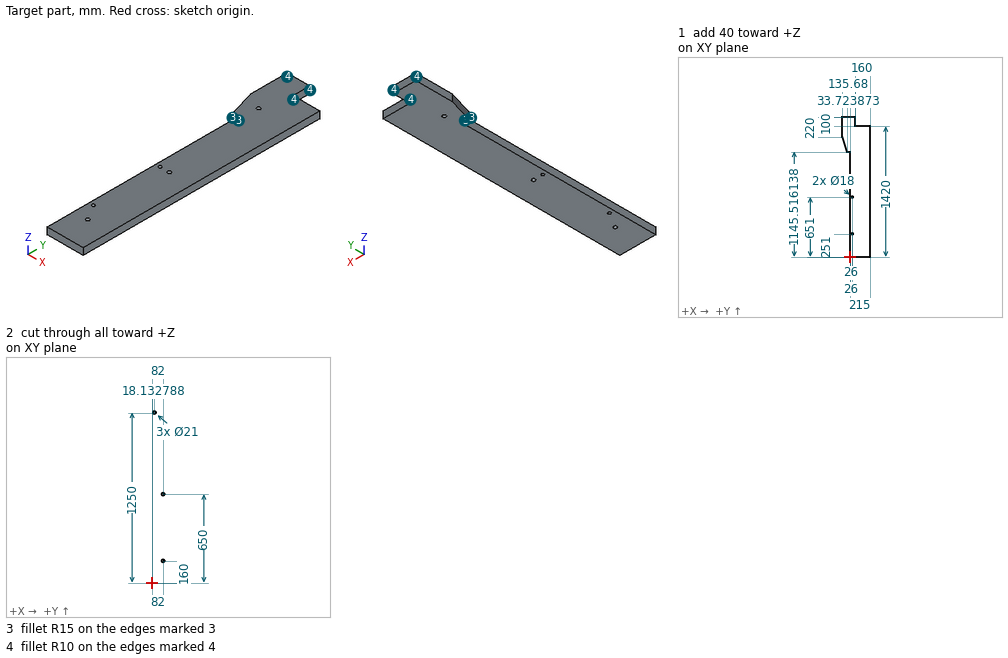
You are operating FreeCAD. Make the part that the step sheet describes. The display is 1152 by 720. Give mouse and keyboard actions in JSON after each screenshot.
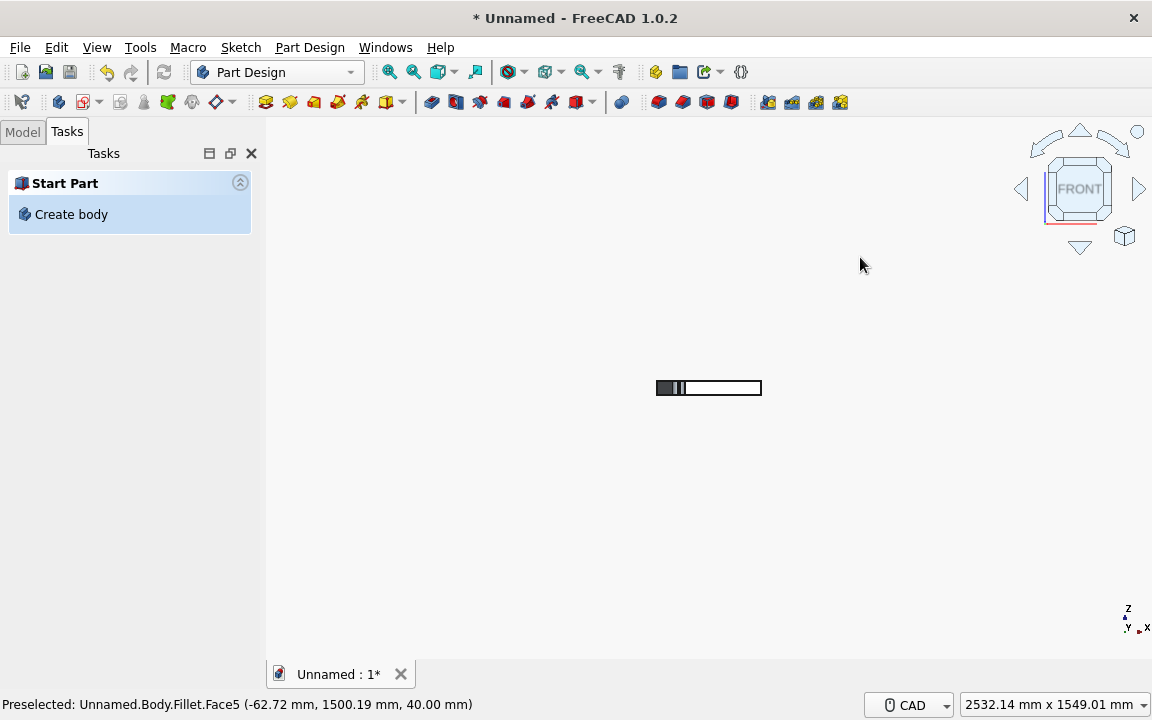
{"action": "key", "text": "v f"}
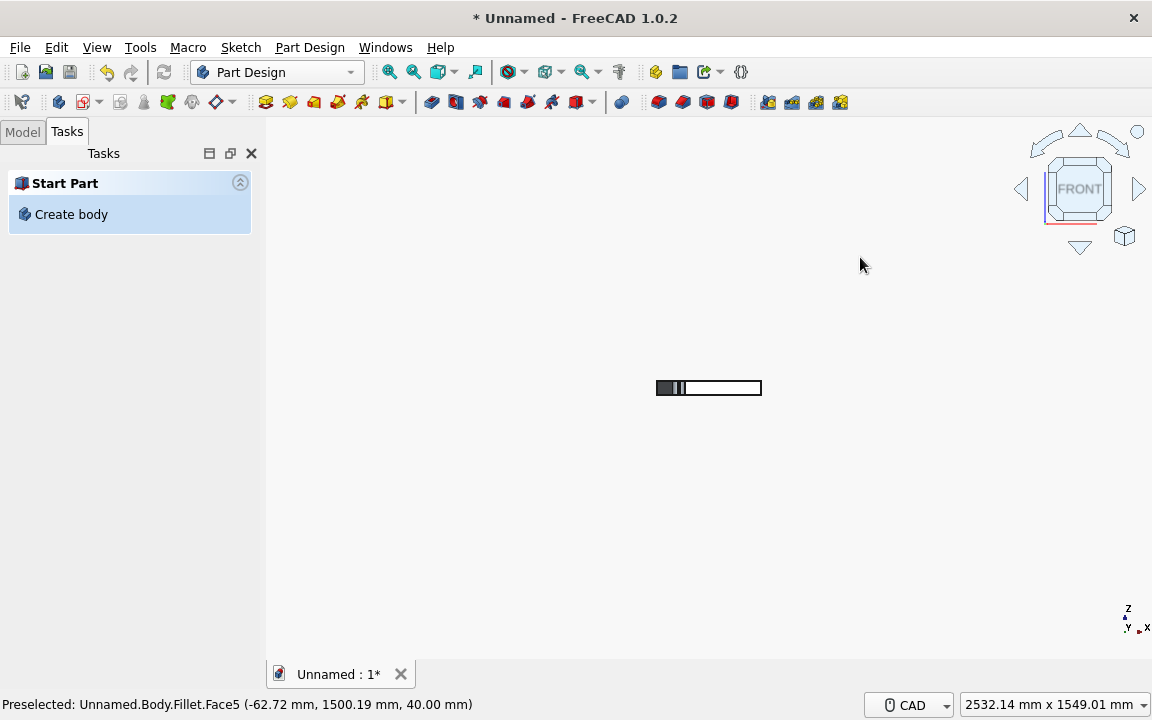
{"action": "scroll", "coordinate": [657, 387], "scroll_direction": "up", "scroll_amount": 6}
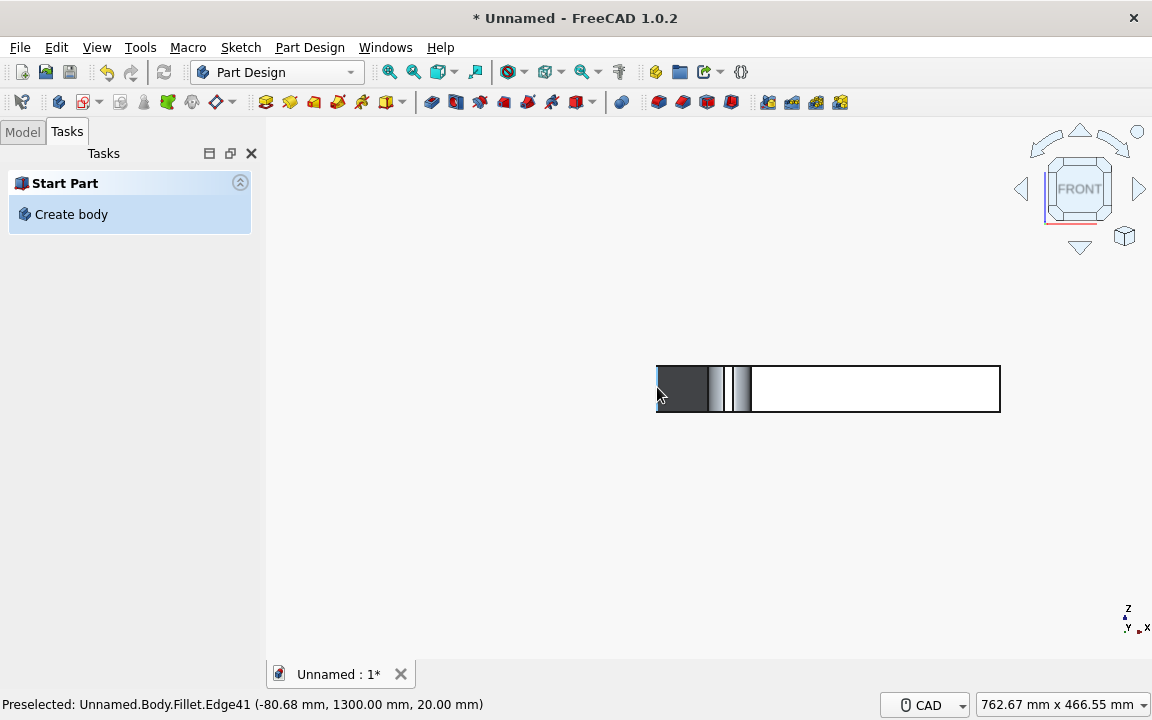
{"action": "key", "text": "v f"}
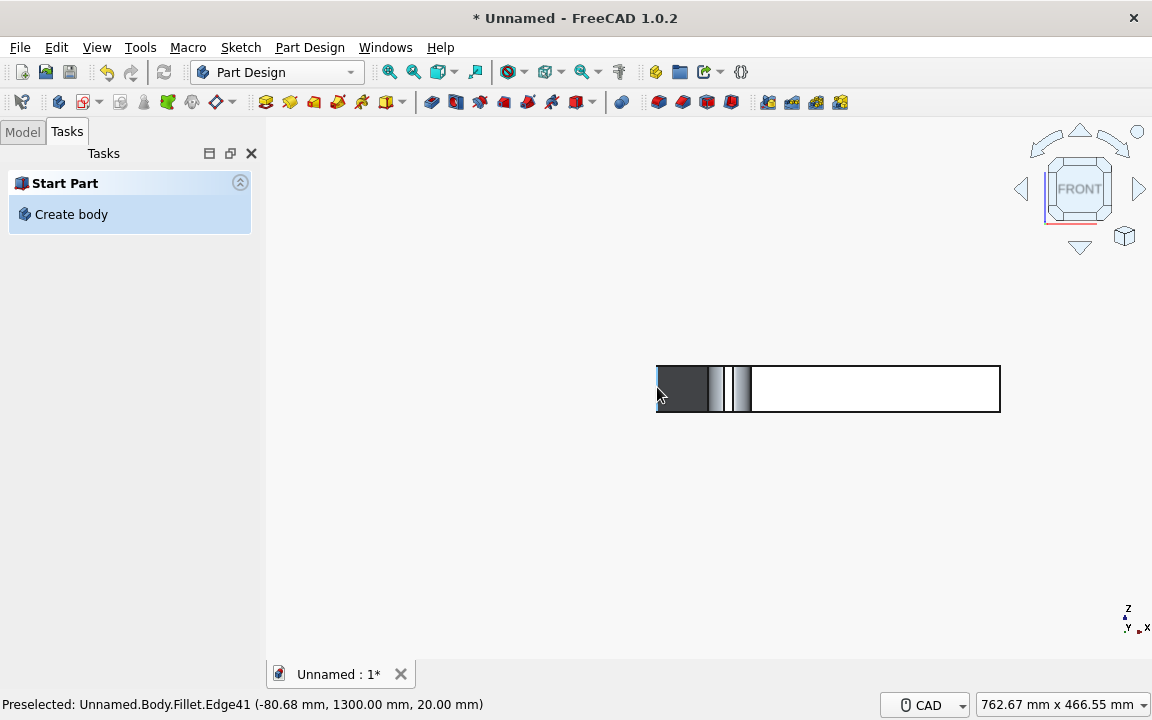
{"action": "key", "text": "3"}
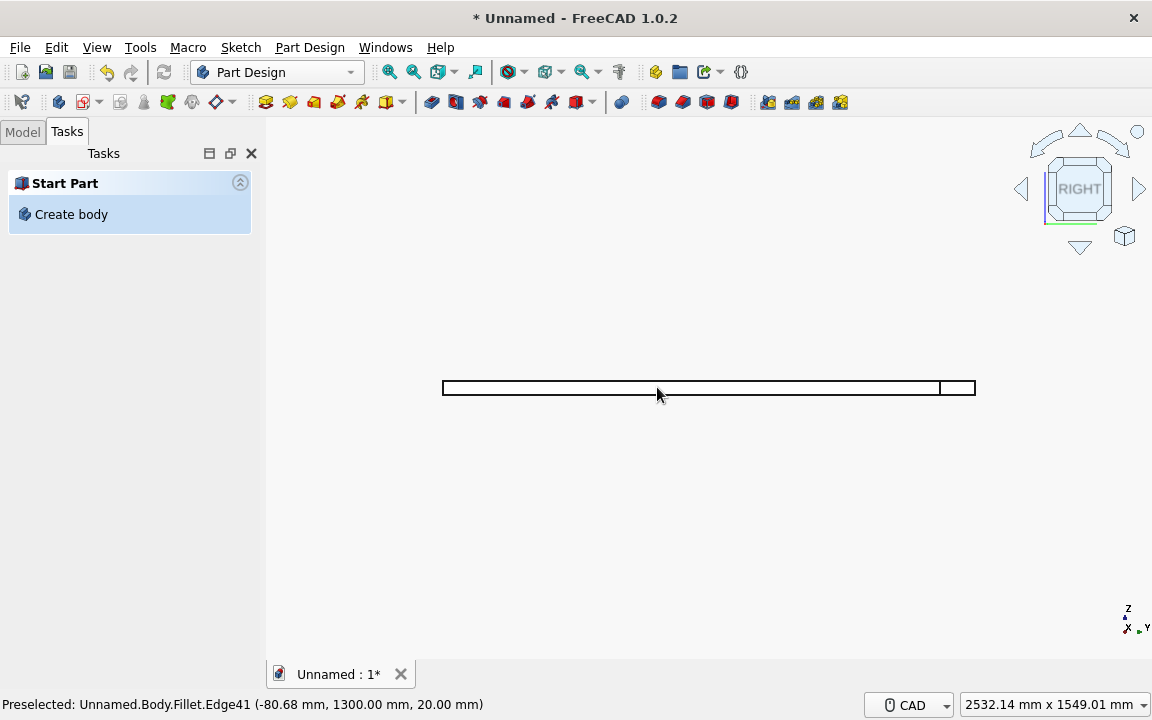
{"action": "left_click", "coordinate": [975, 387]}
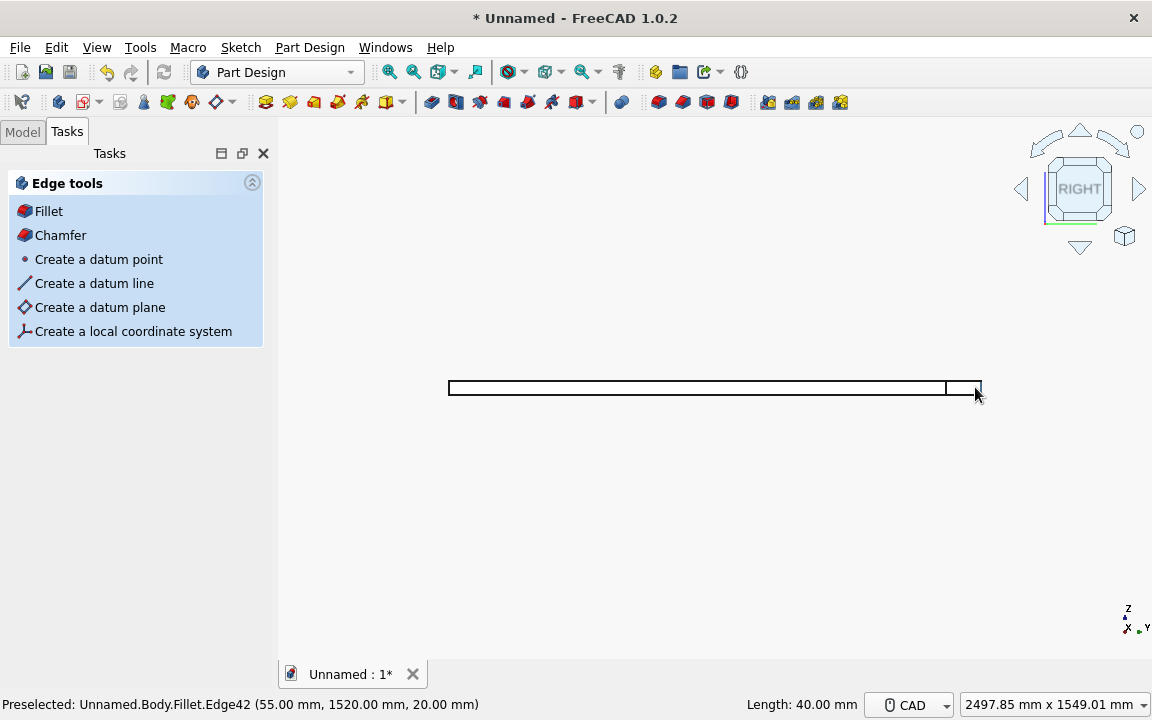
{"action": "scroll", "coordinate": [981, 387], "scroll_direction": "up", "scroll_amount": 6}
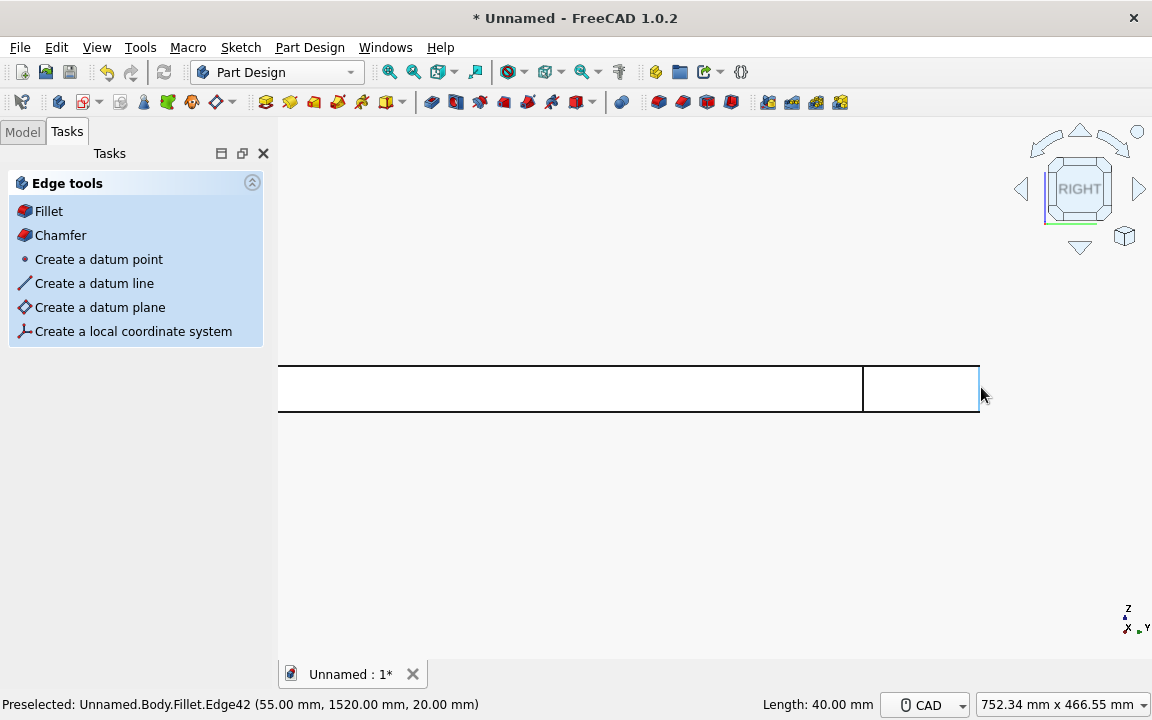
{"action": "key", "text": "v f"}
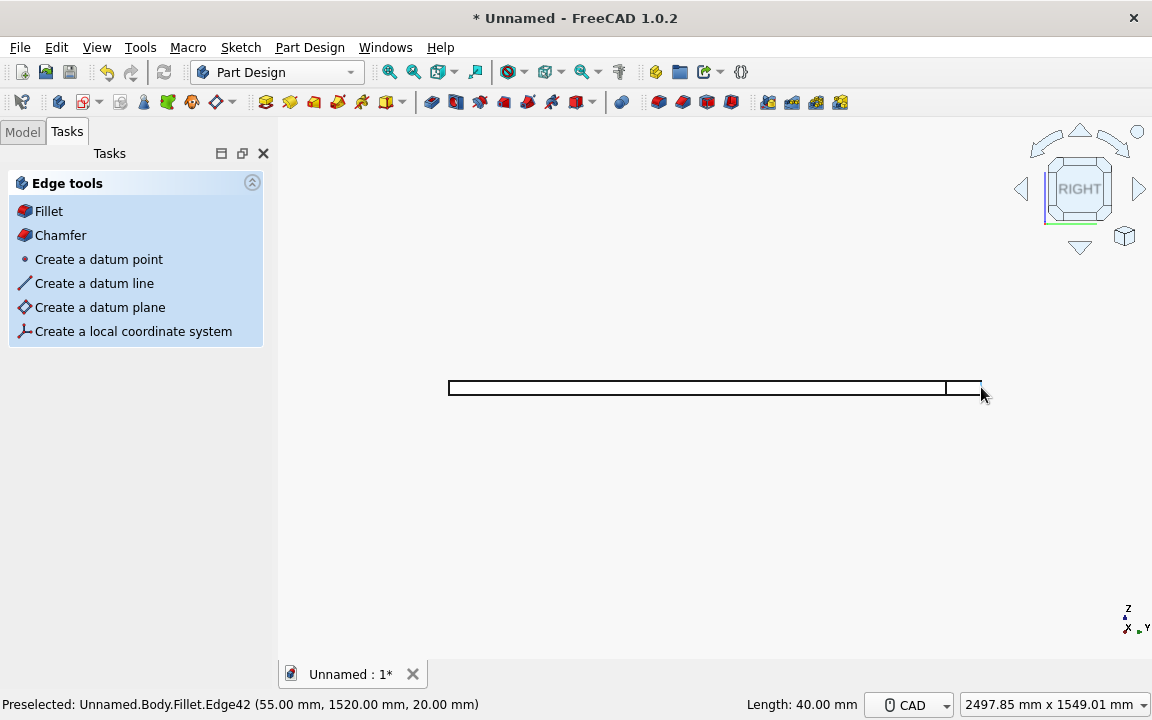
{"action": "key", "text": "5"}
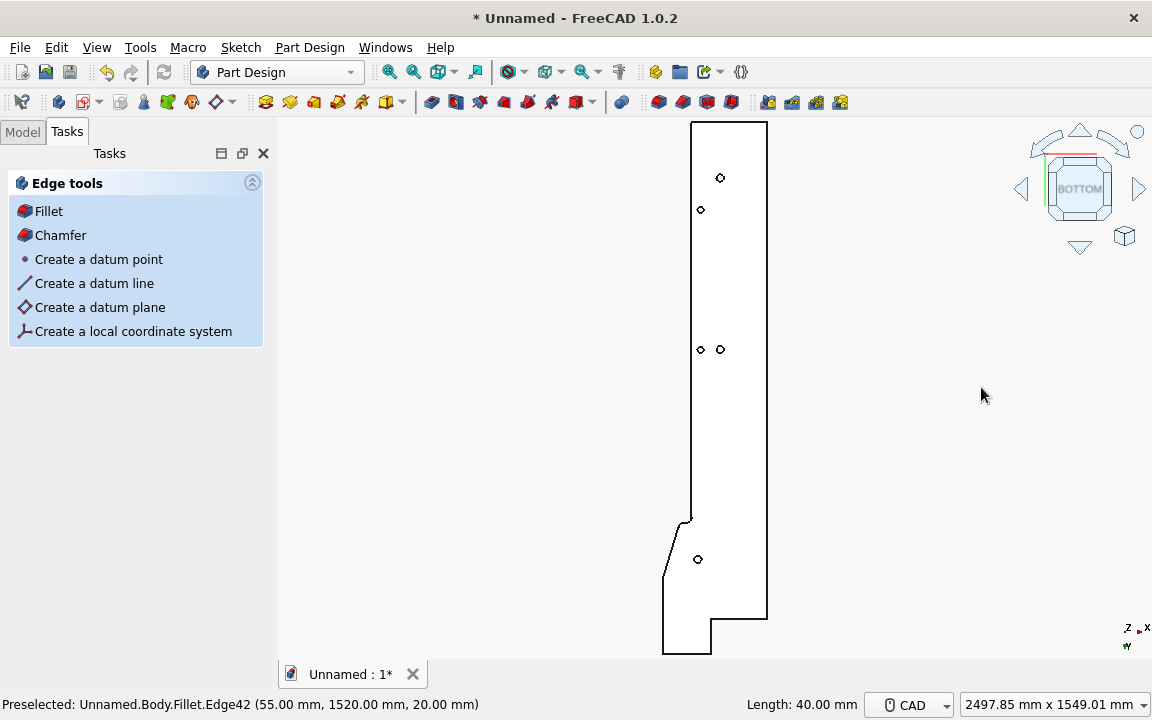
{"action": "key", "text": "4"}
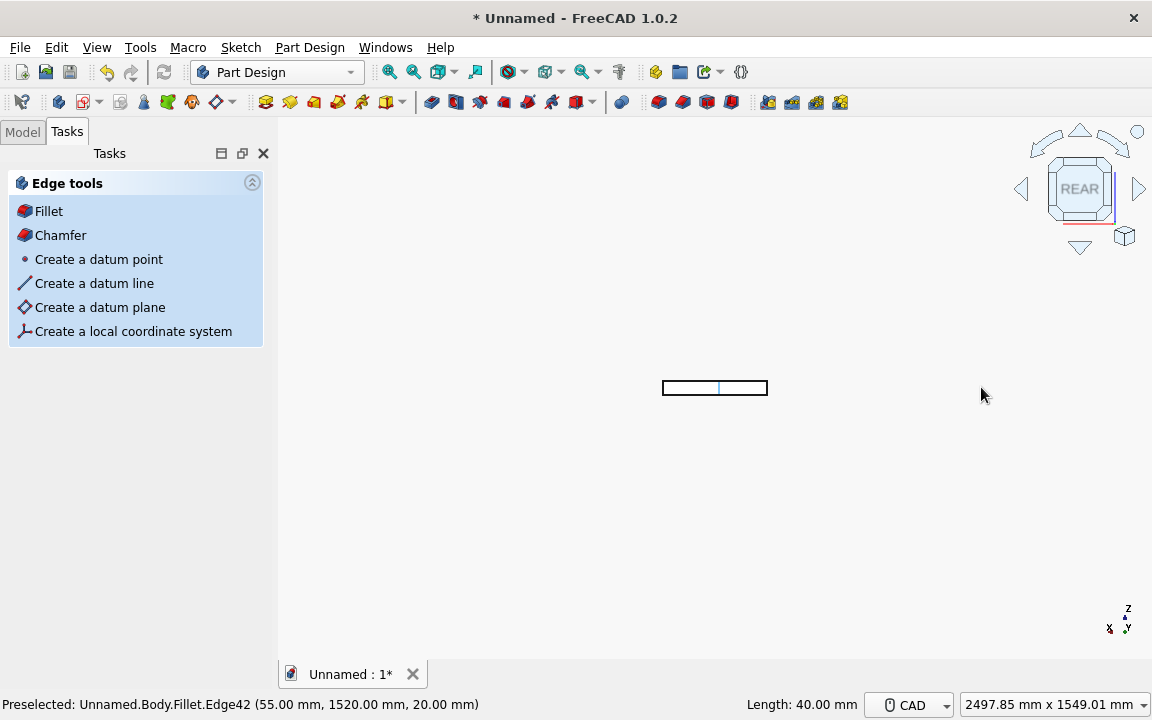
{"action": "key", "text": "v f"}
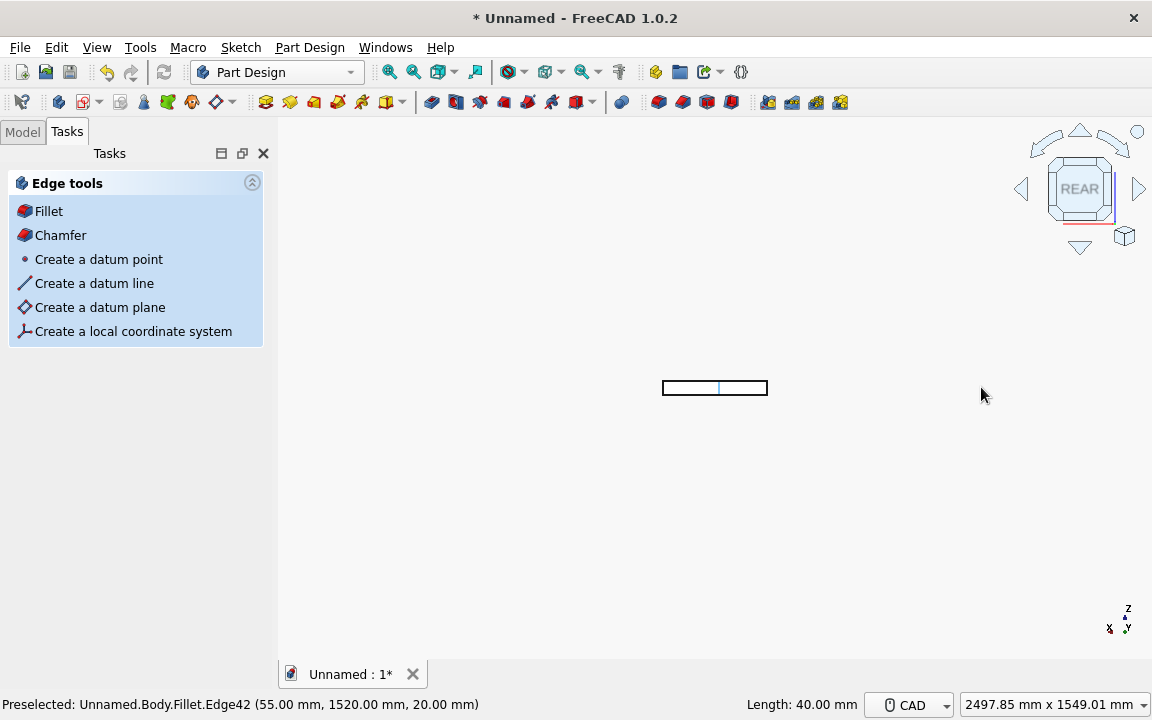
{"action": "left_click", "coordinate": [767, 387], "text": "ctrl"}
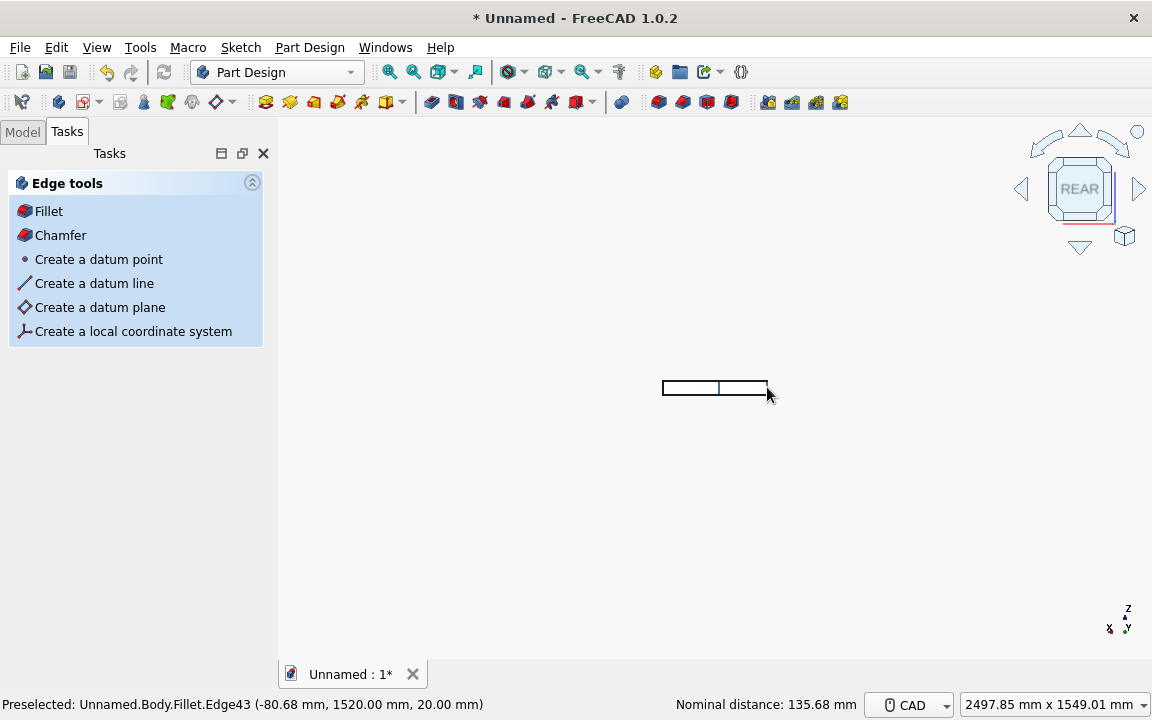
{"action": "scroll", "coordinate": [719, 387], "scroll_direction": "up", "scroll_amount": 6}